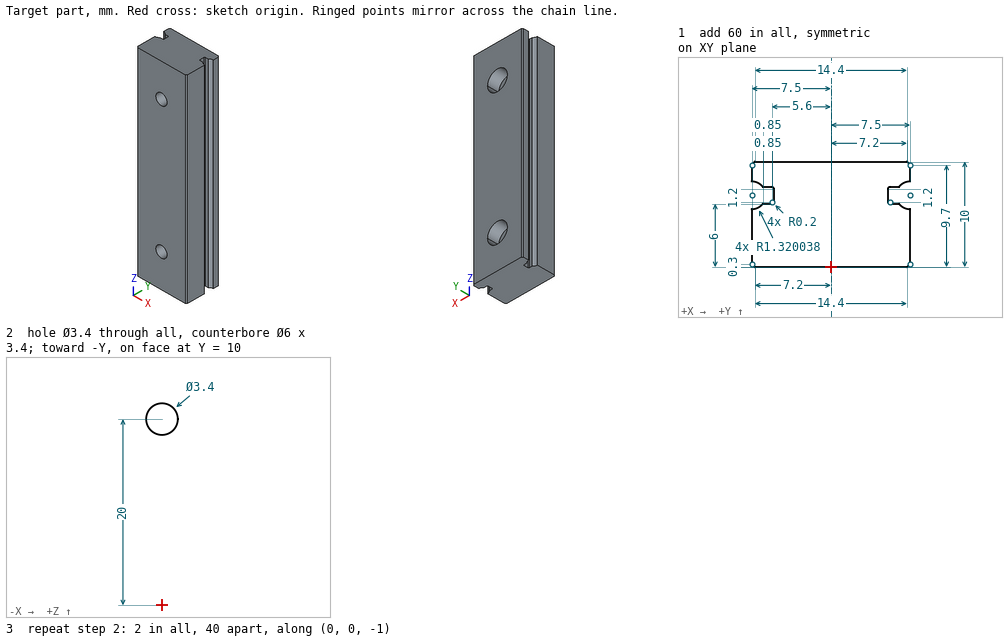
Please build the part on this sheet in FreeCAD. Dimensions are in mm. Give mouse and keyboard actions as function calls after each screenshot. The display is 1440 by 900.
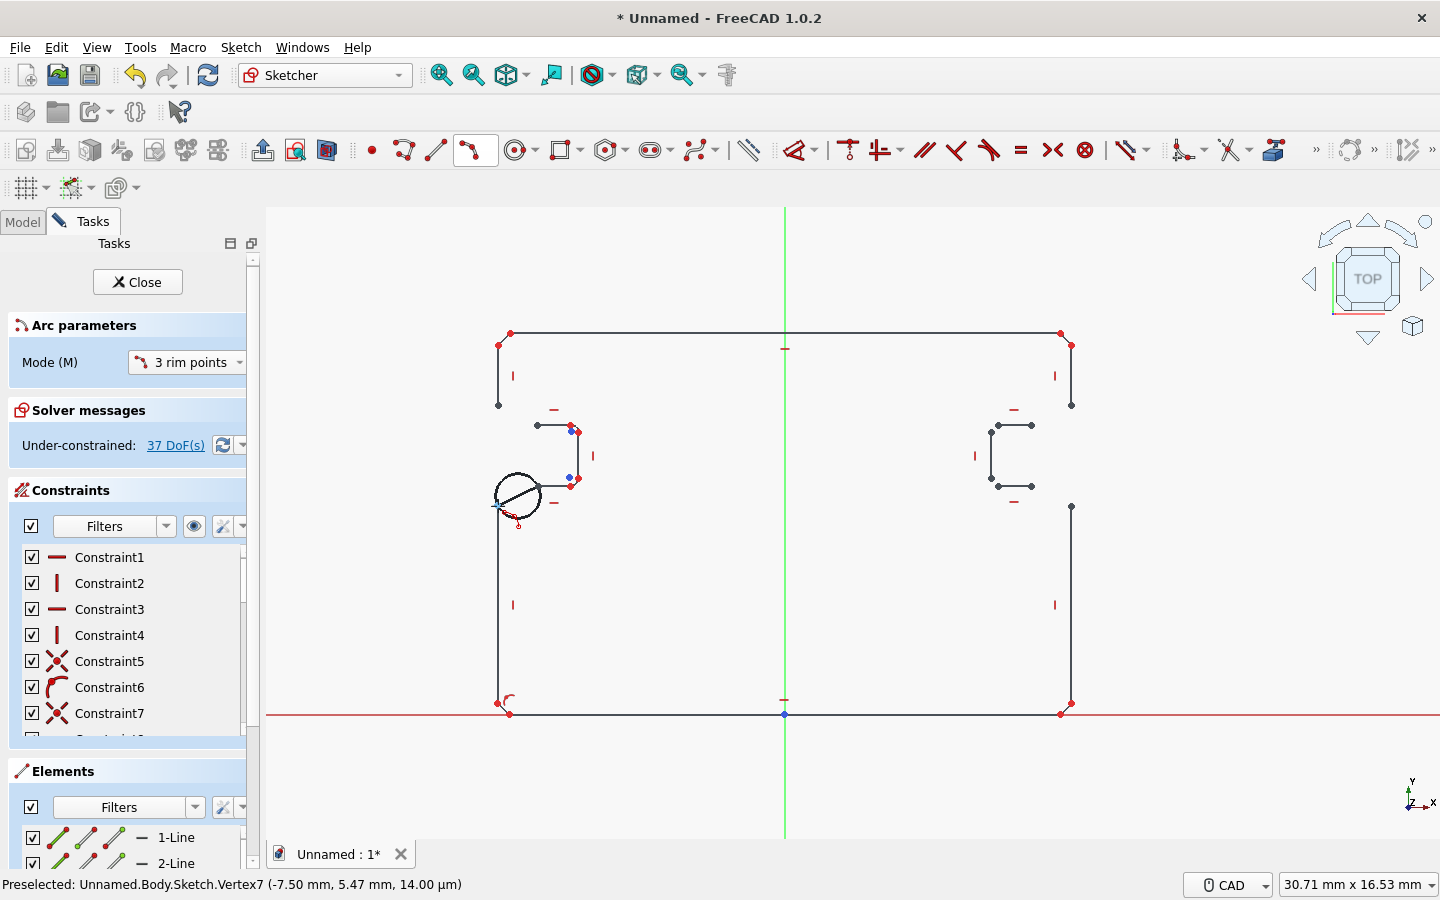
scroll(520, 500, up, 6)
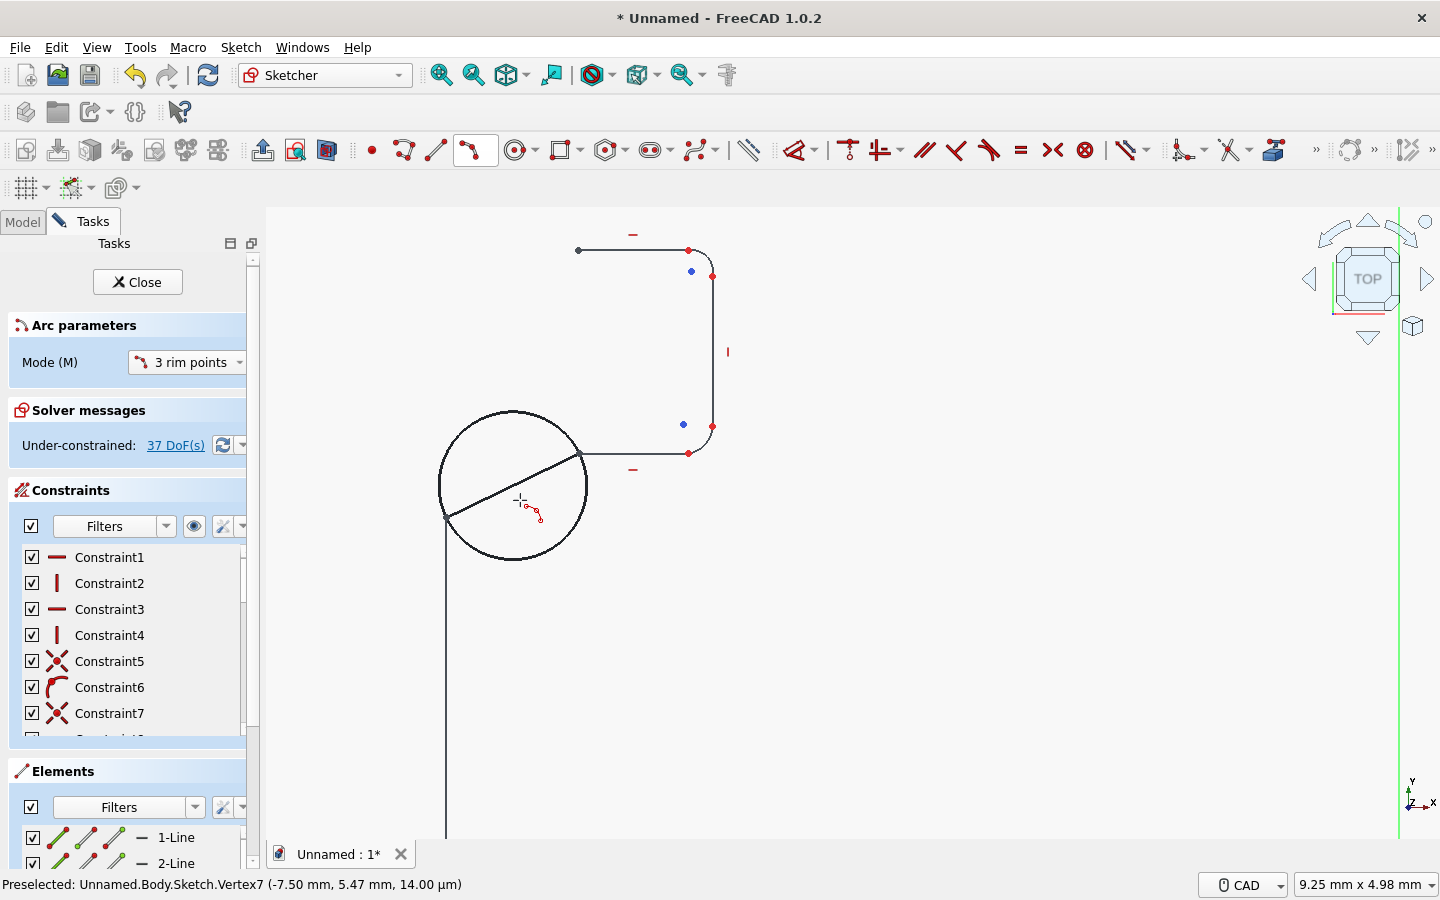
click(521, 499)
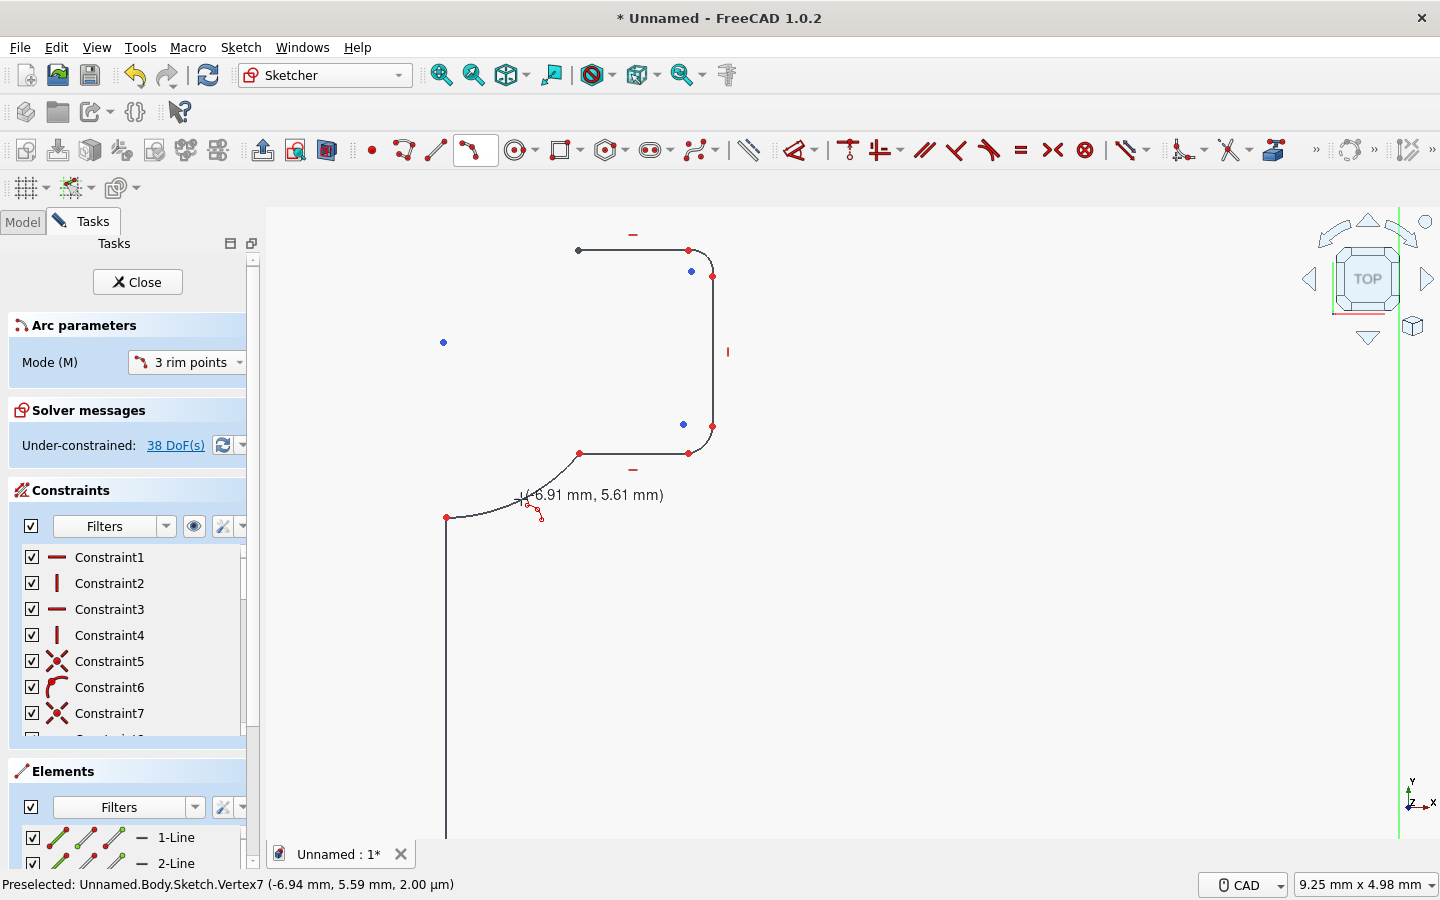
scroll(520, 499, down, 6)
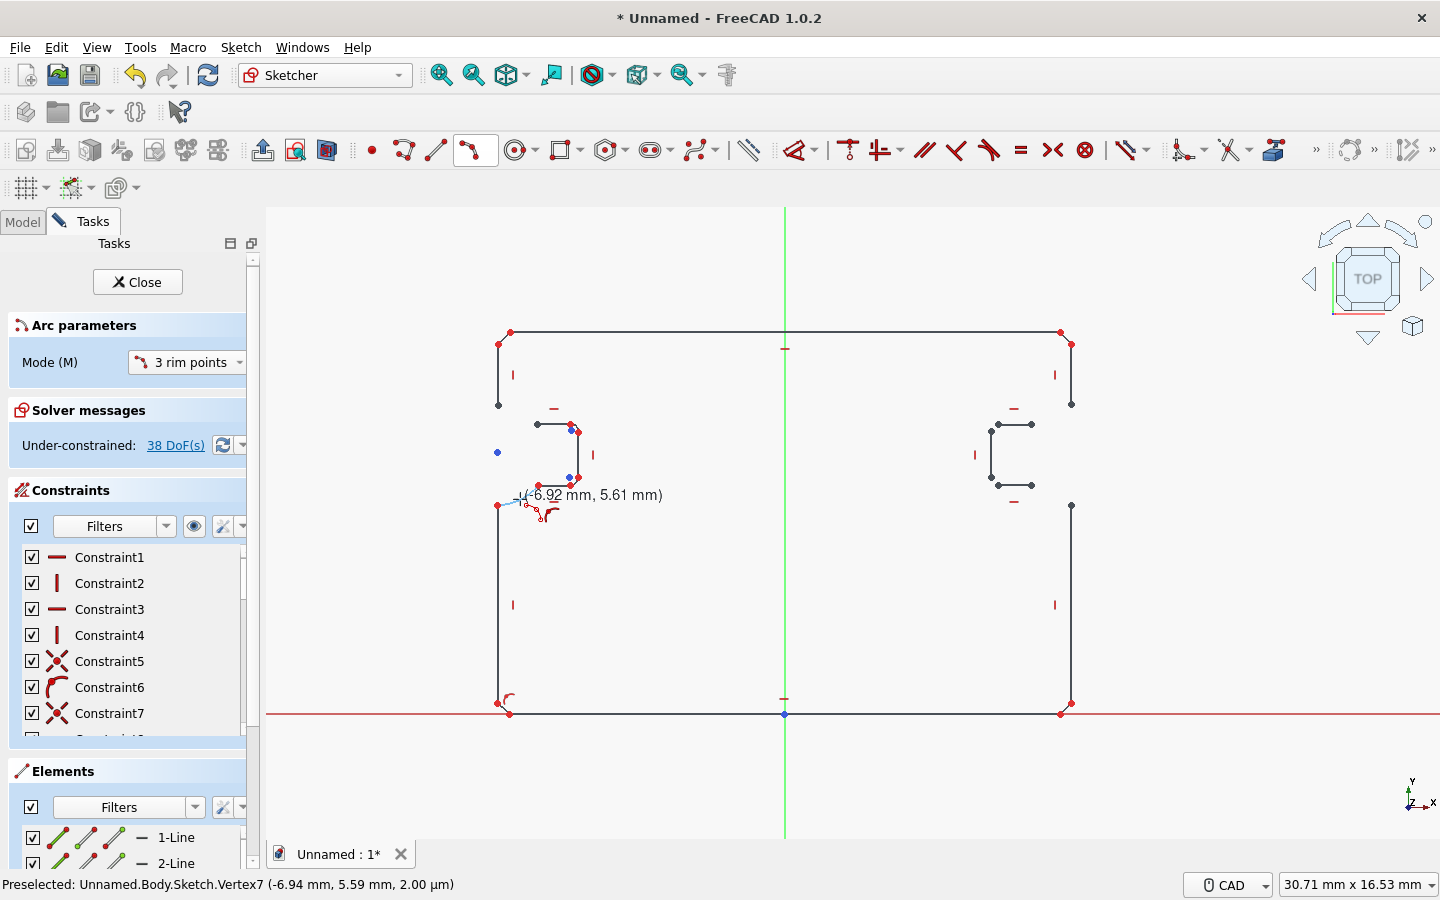
click(1071, 505)
click(1031, 485)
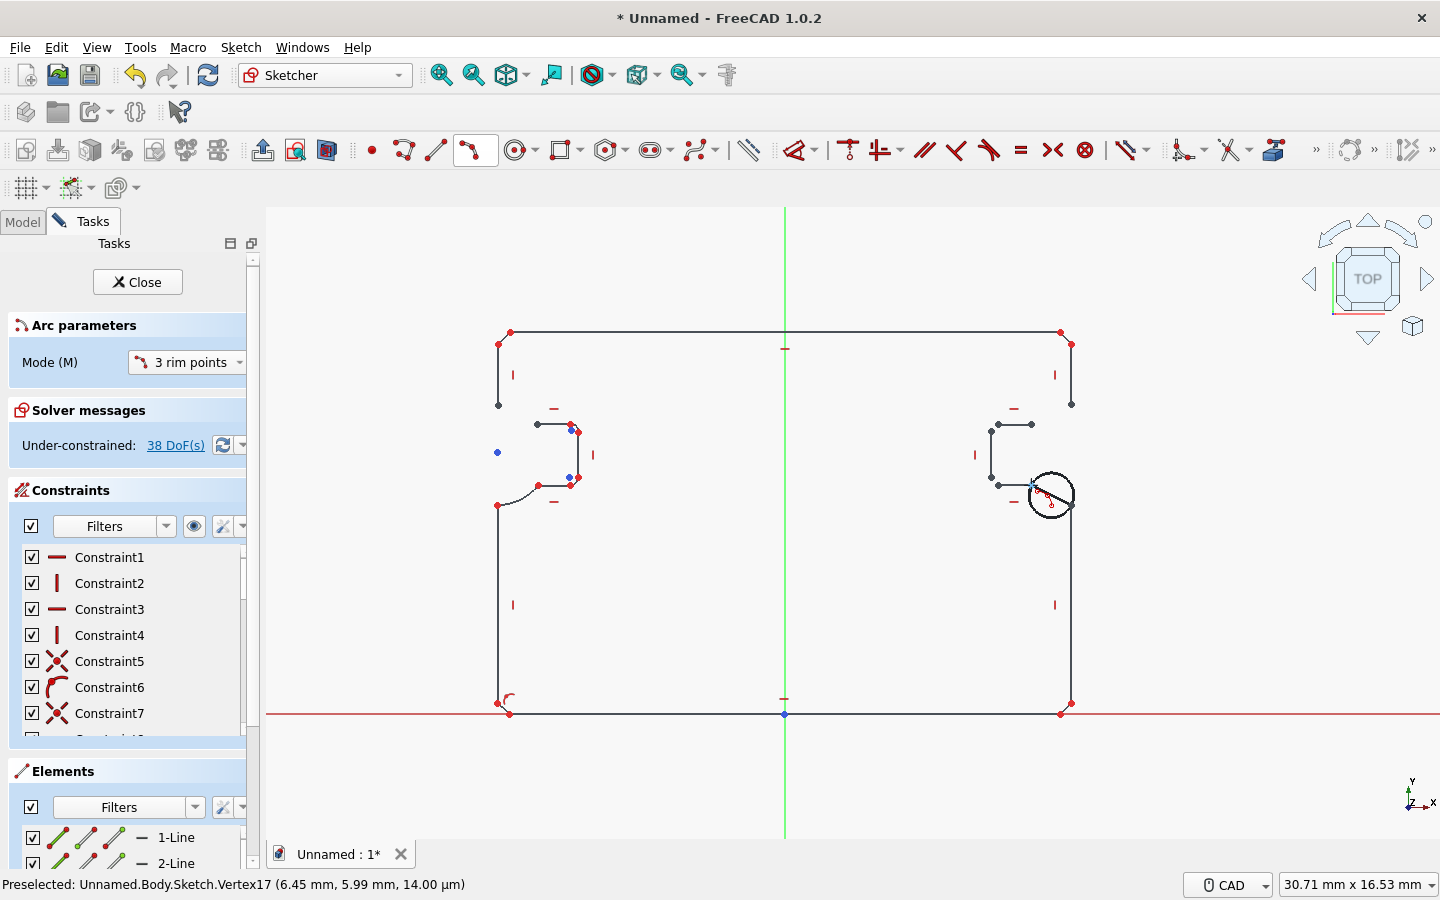
scroll(1049, 499, up, 6)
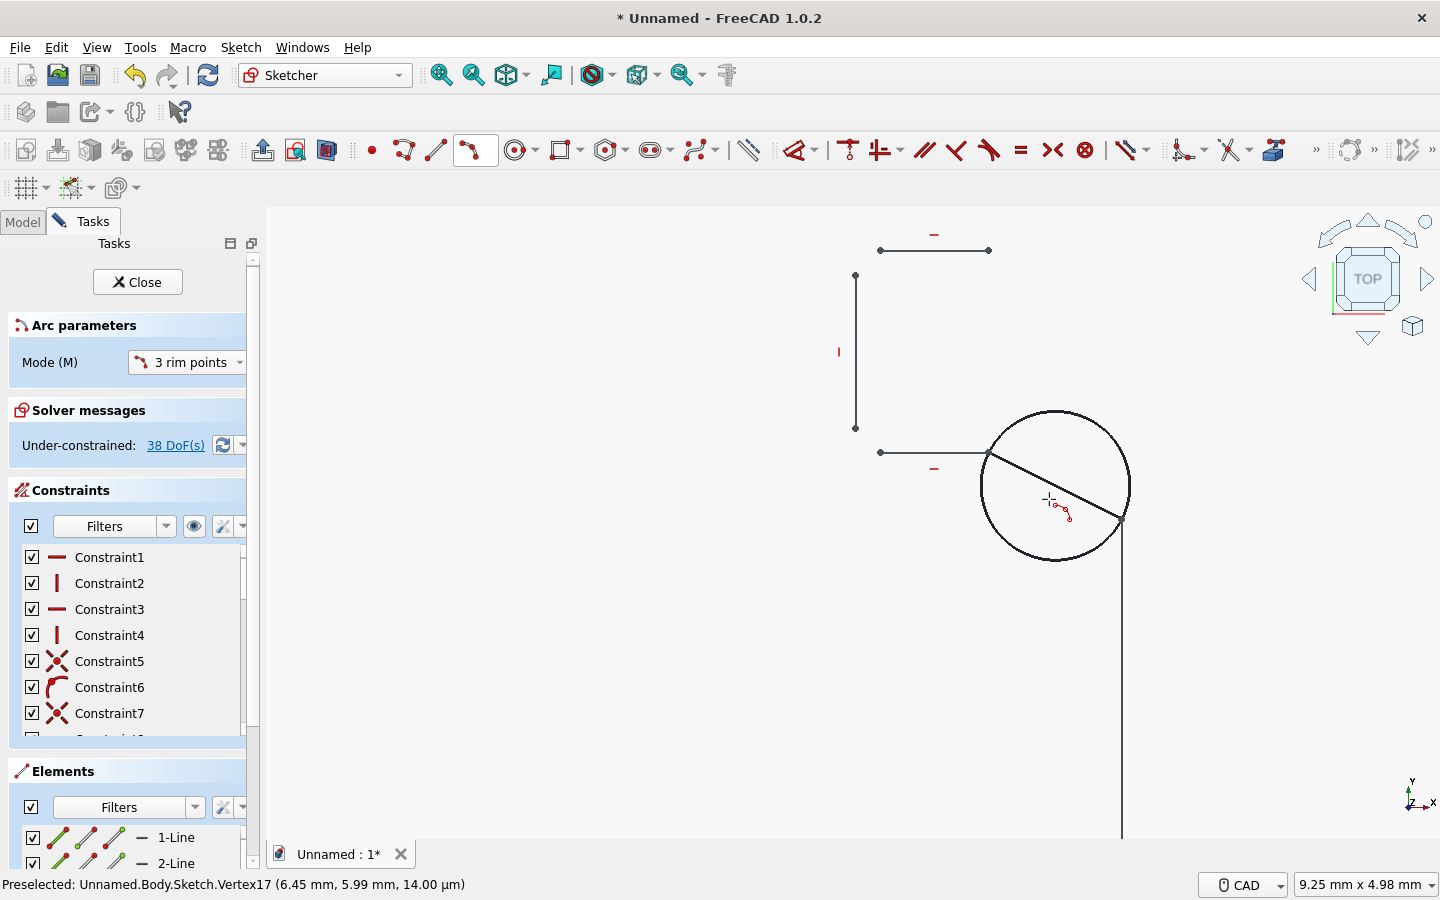
click(1048, 499)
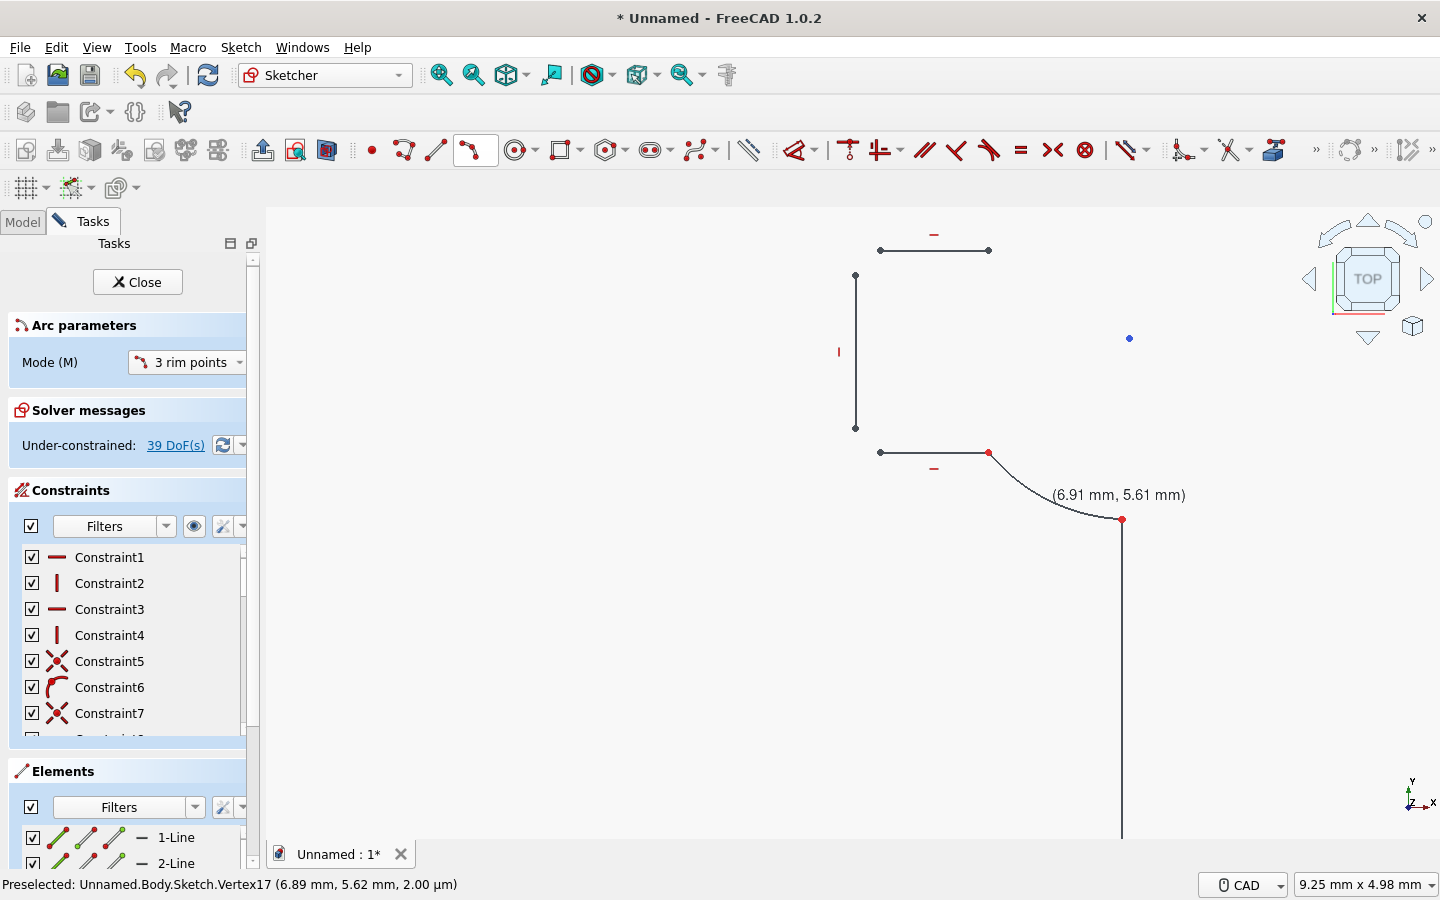
click(880, 453)
click(856, 428)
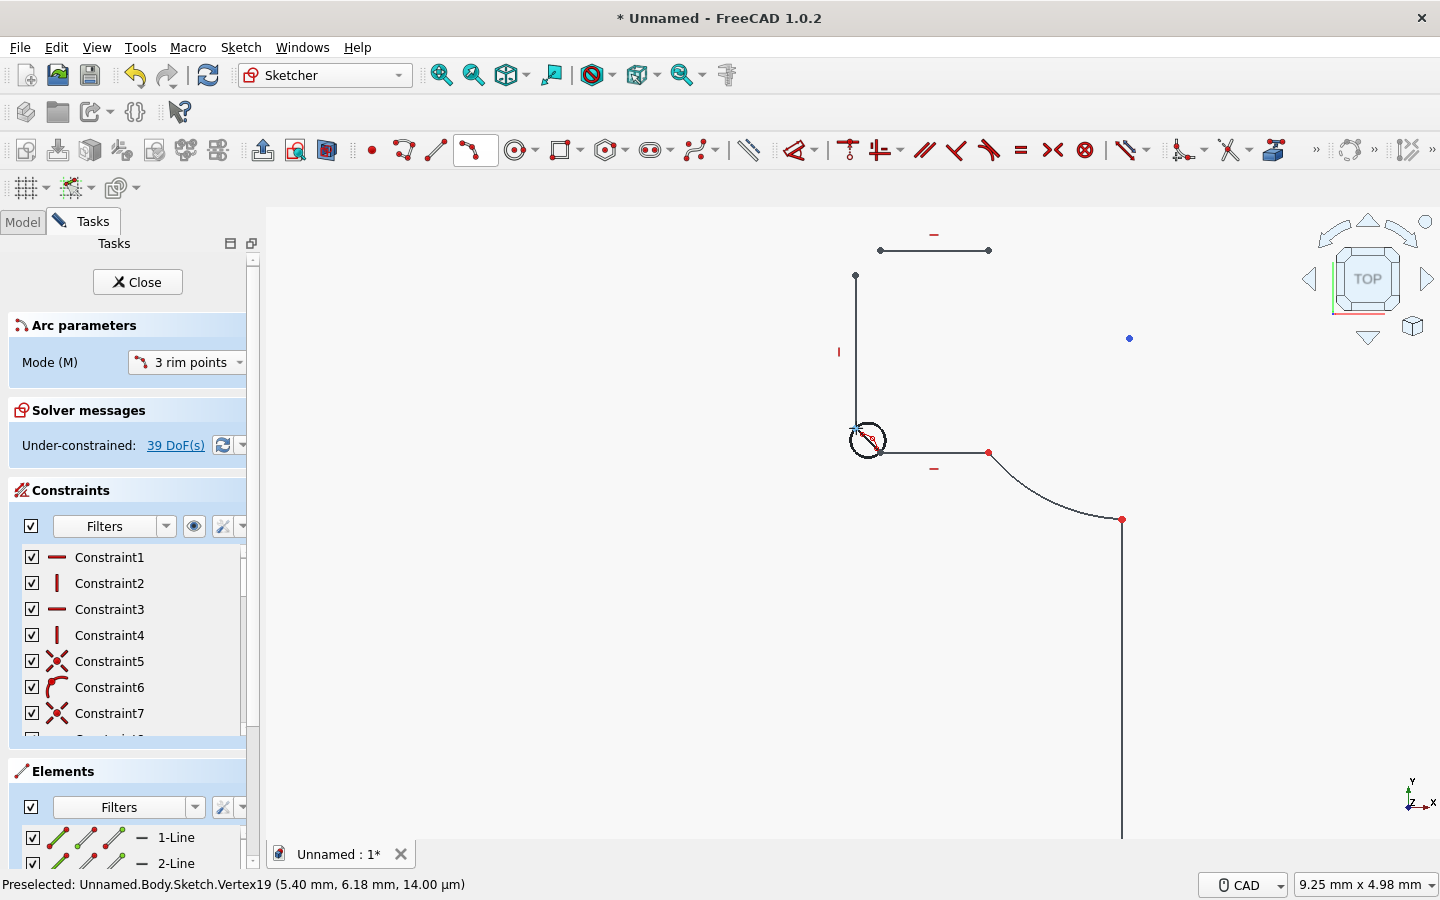
scroll(863, 443, up, 4)